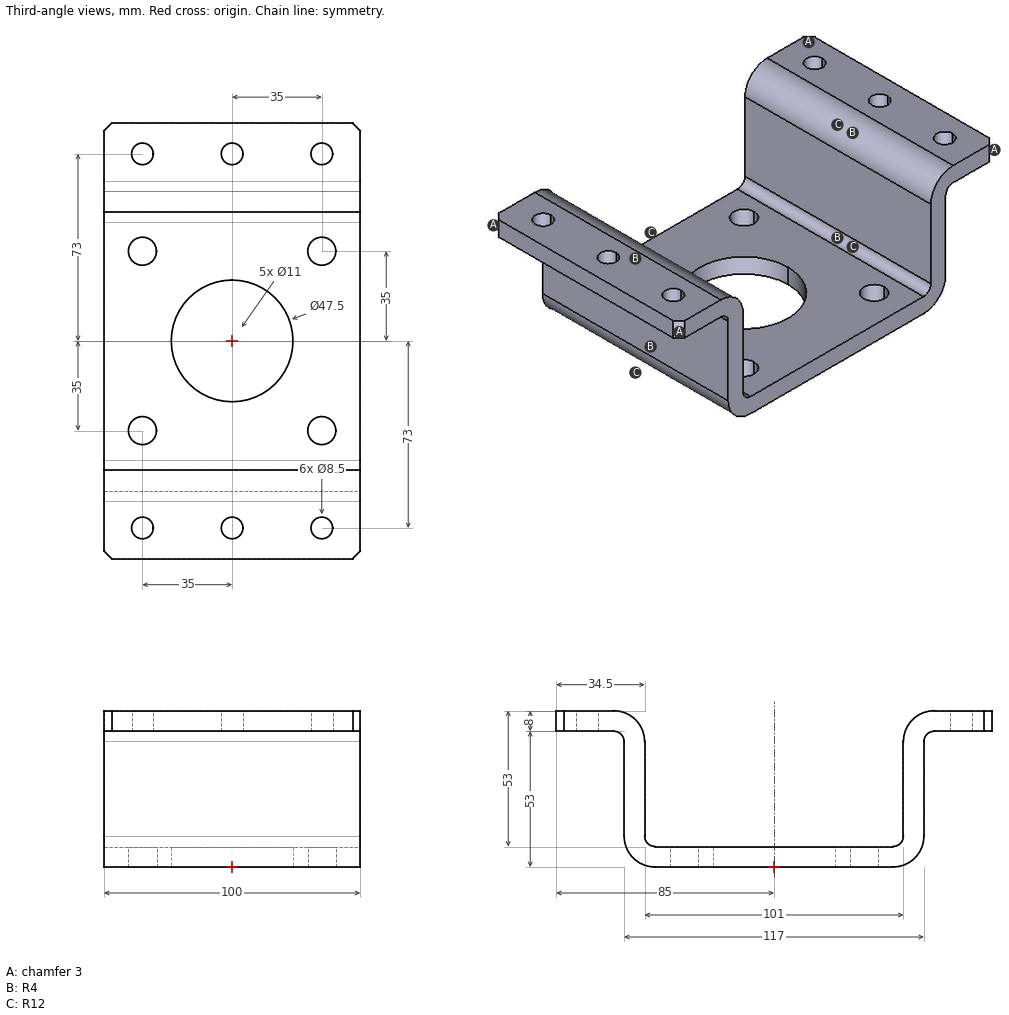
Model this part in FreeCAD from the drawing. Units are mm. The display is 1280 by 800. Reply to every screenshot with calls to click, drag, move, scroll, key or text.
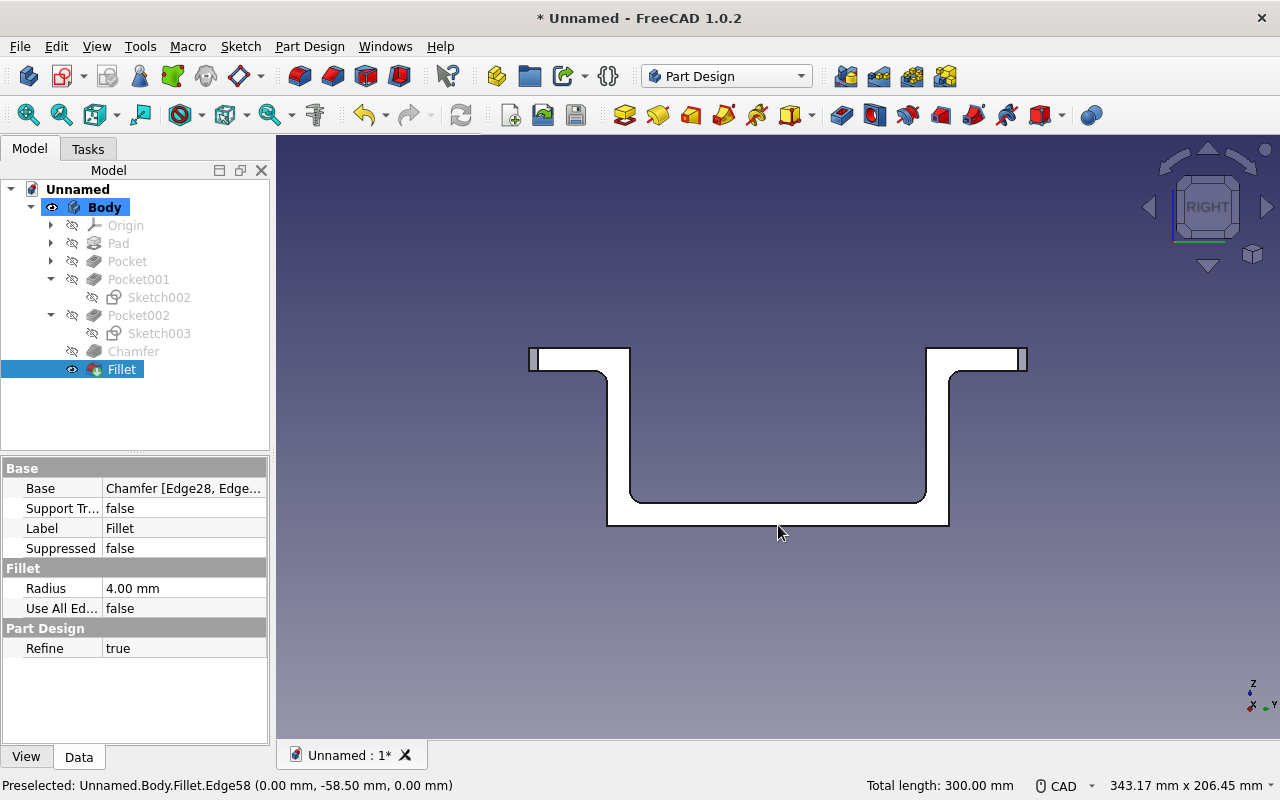
key(5)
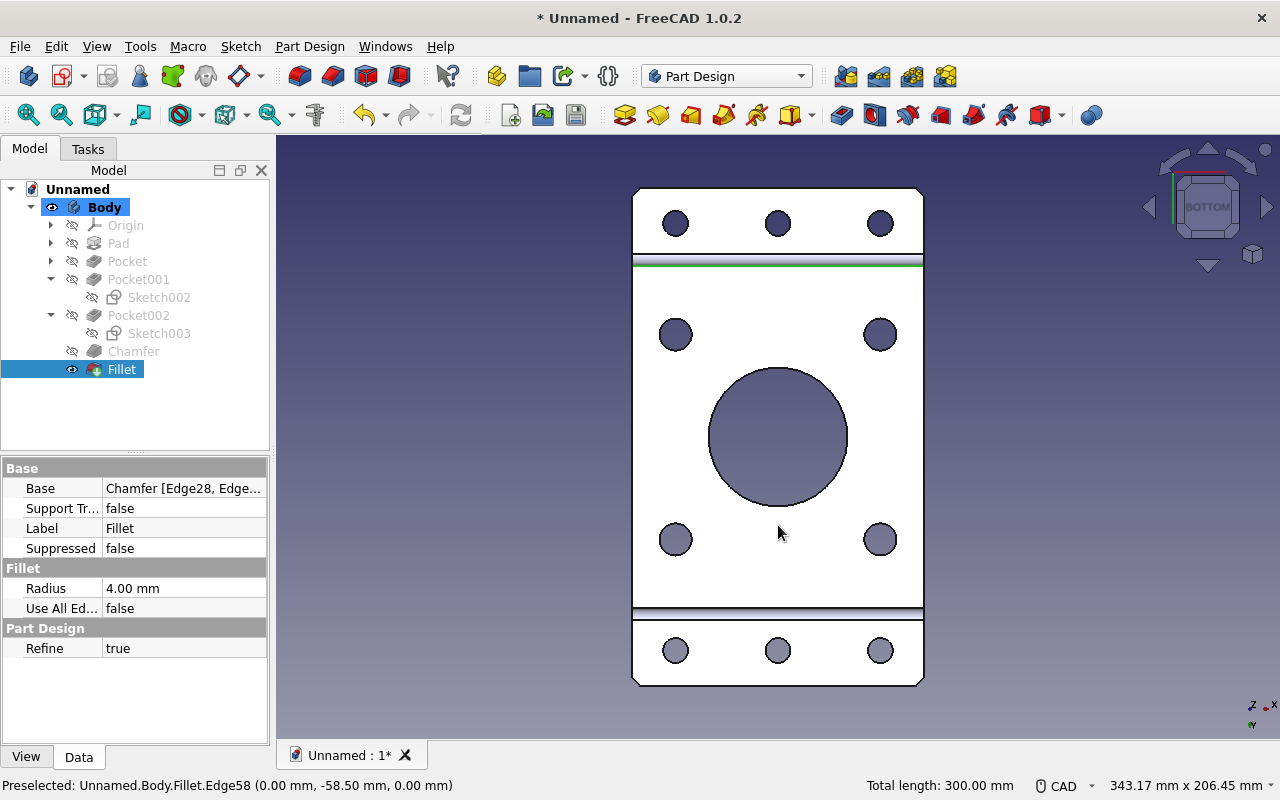
click(778, 607, ctrl)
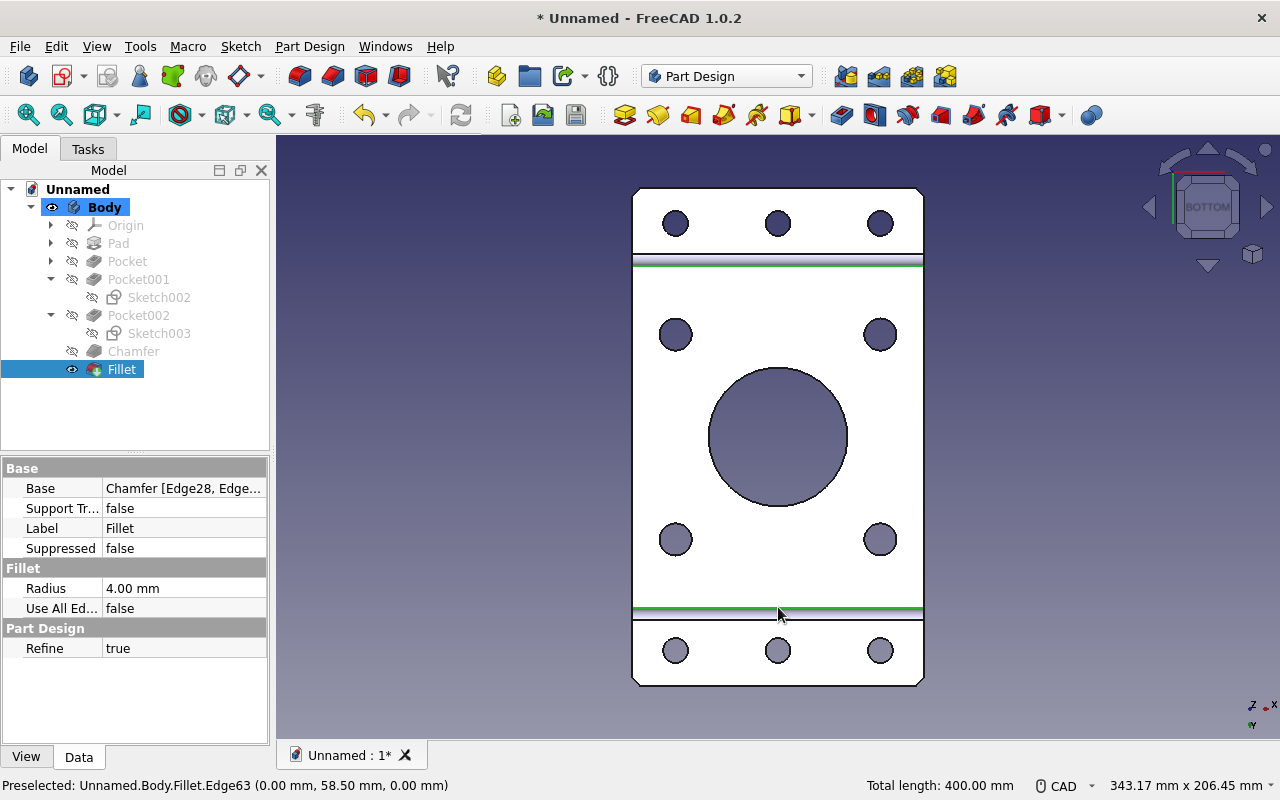
click(300, 76)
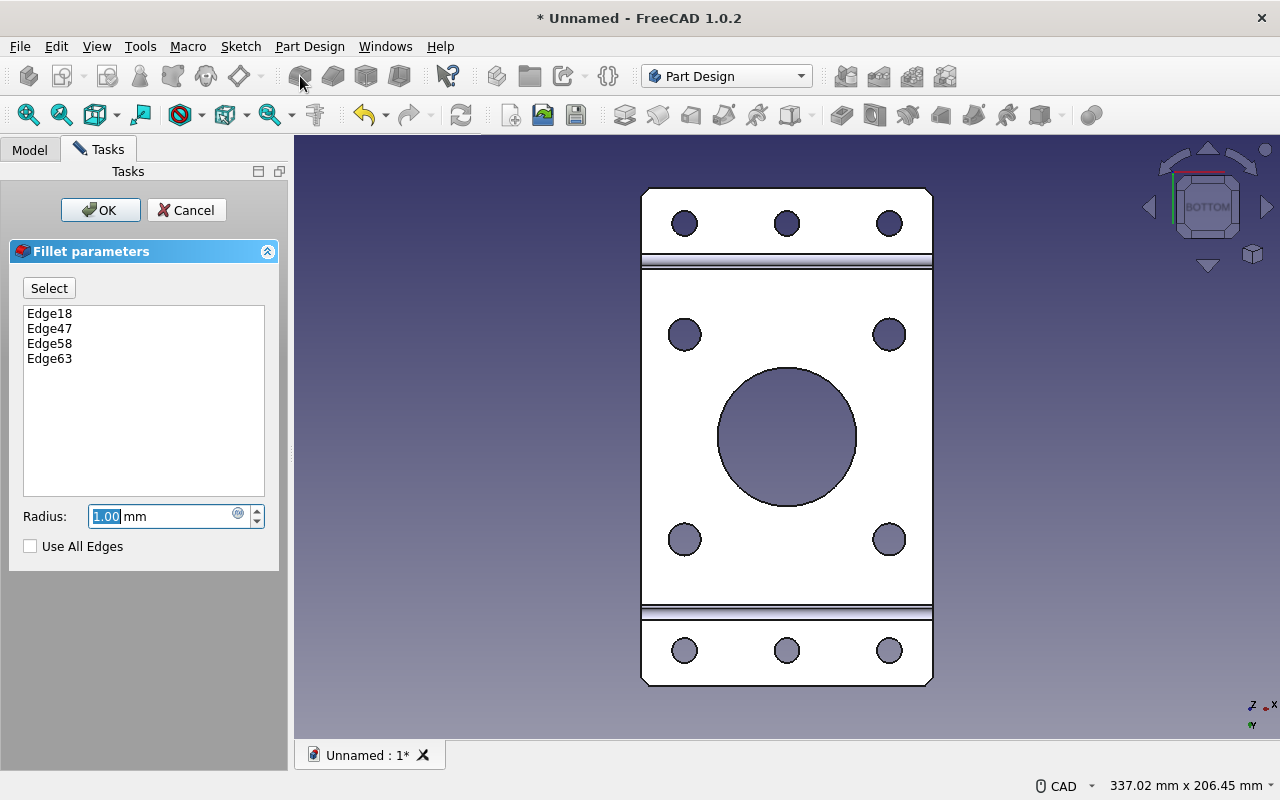
text(12)
key(Tab)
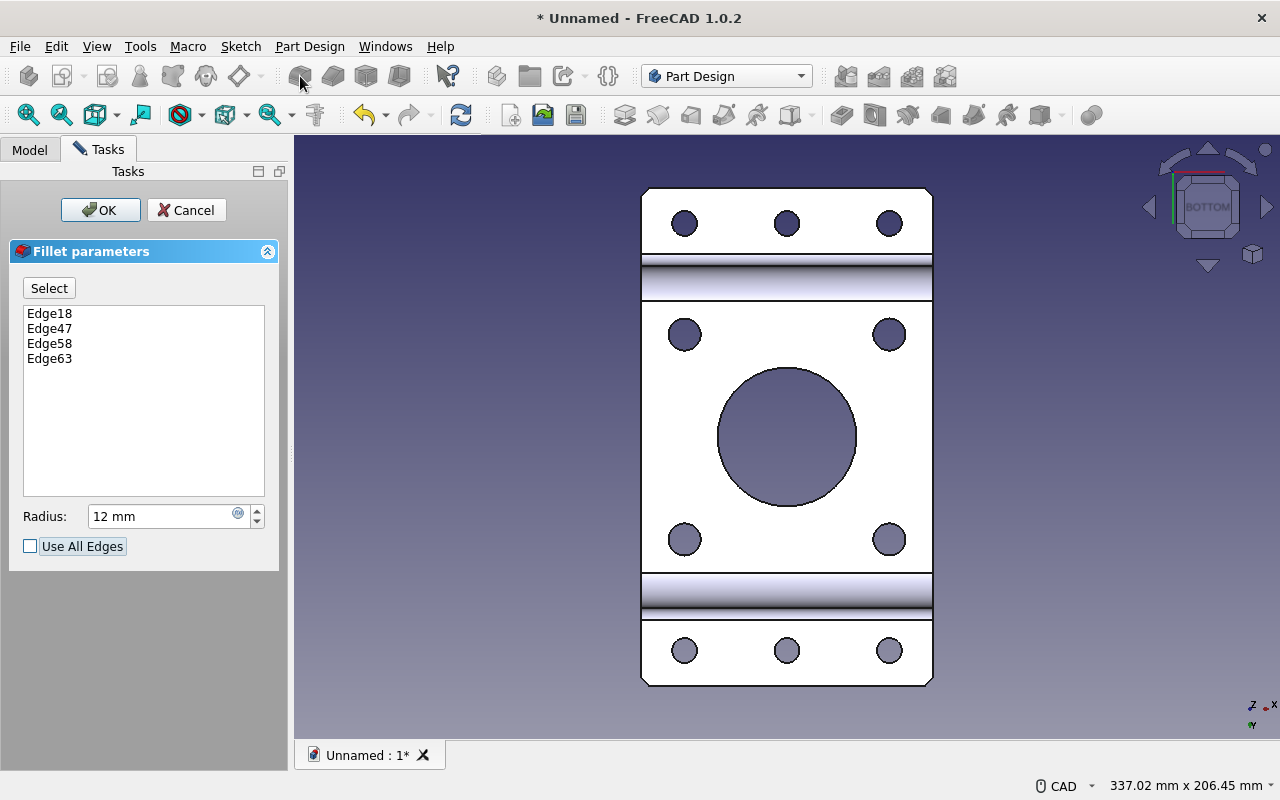
click(101, 210)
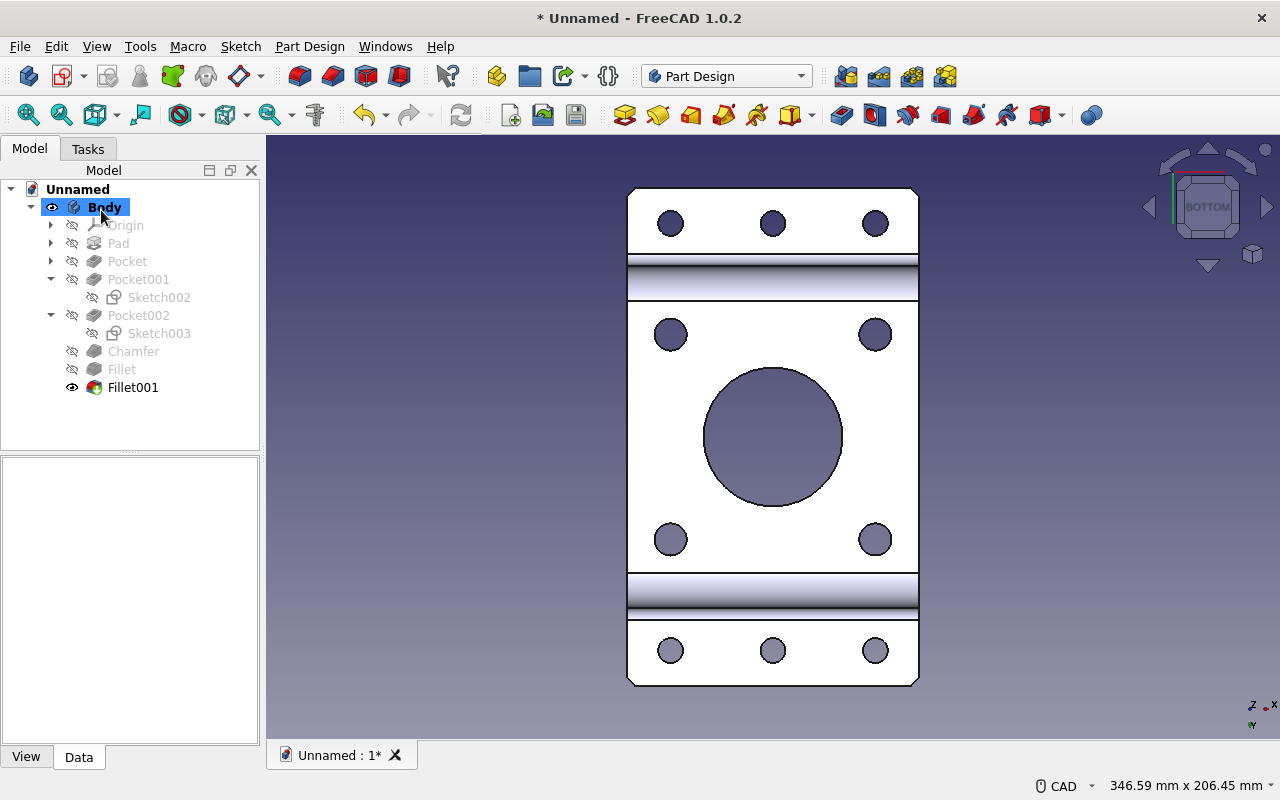
key(0)